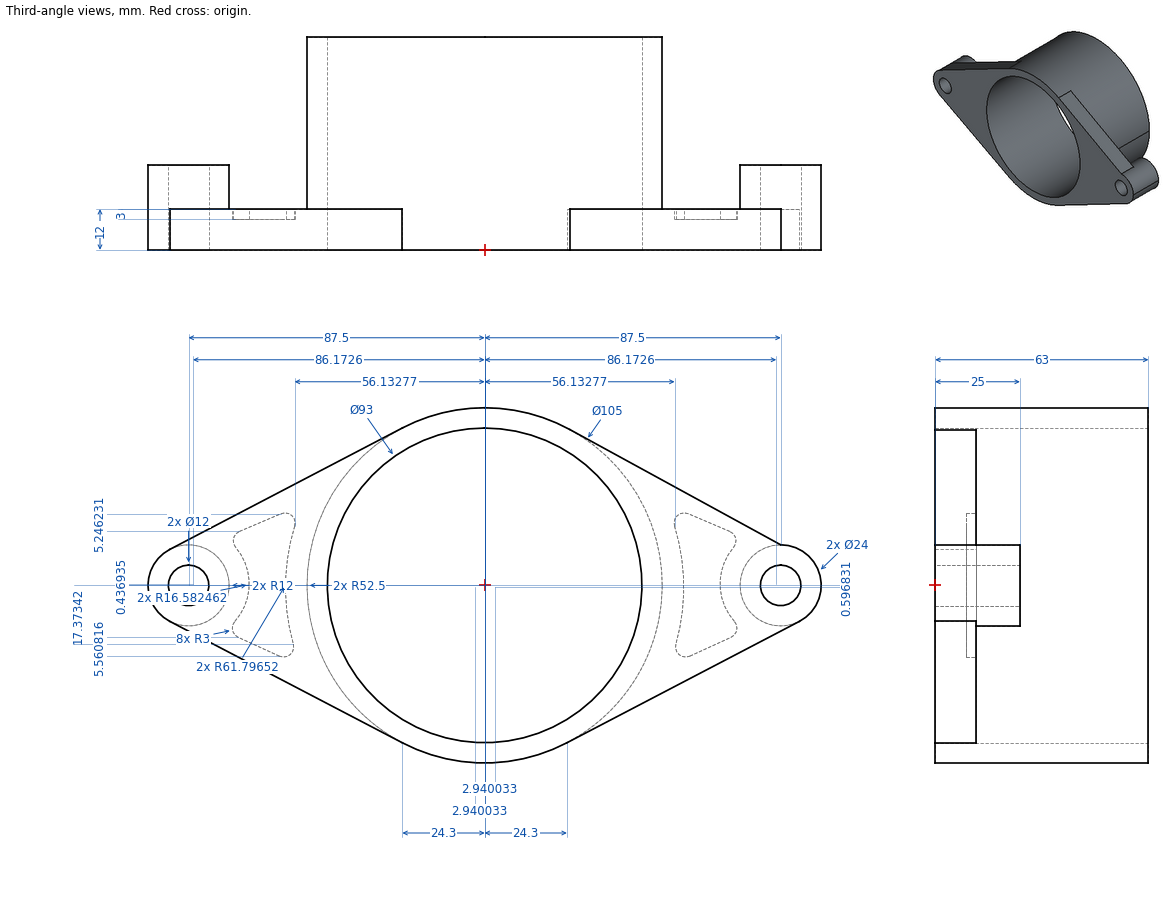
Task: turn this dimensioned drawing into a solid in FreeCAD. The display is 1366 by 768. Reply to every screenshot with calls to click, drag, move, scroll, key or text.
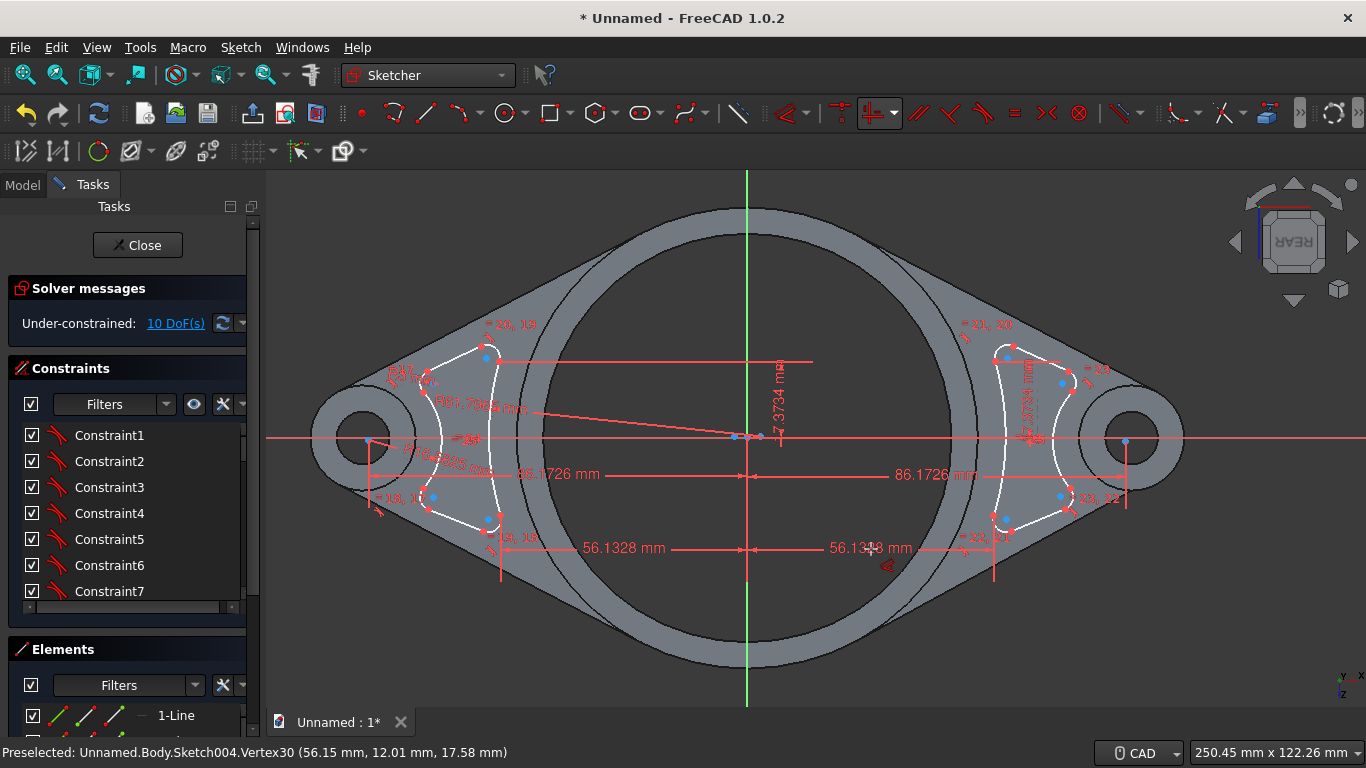
scroll(465, 354, up, 3)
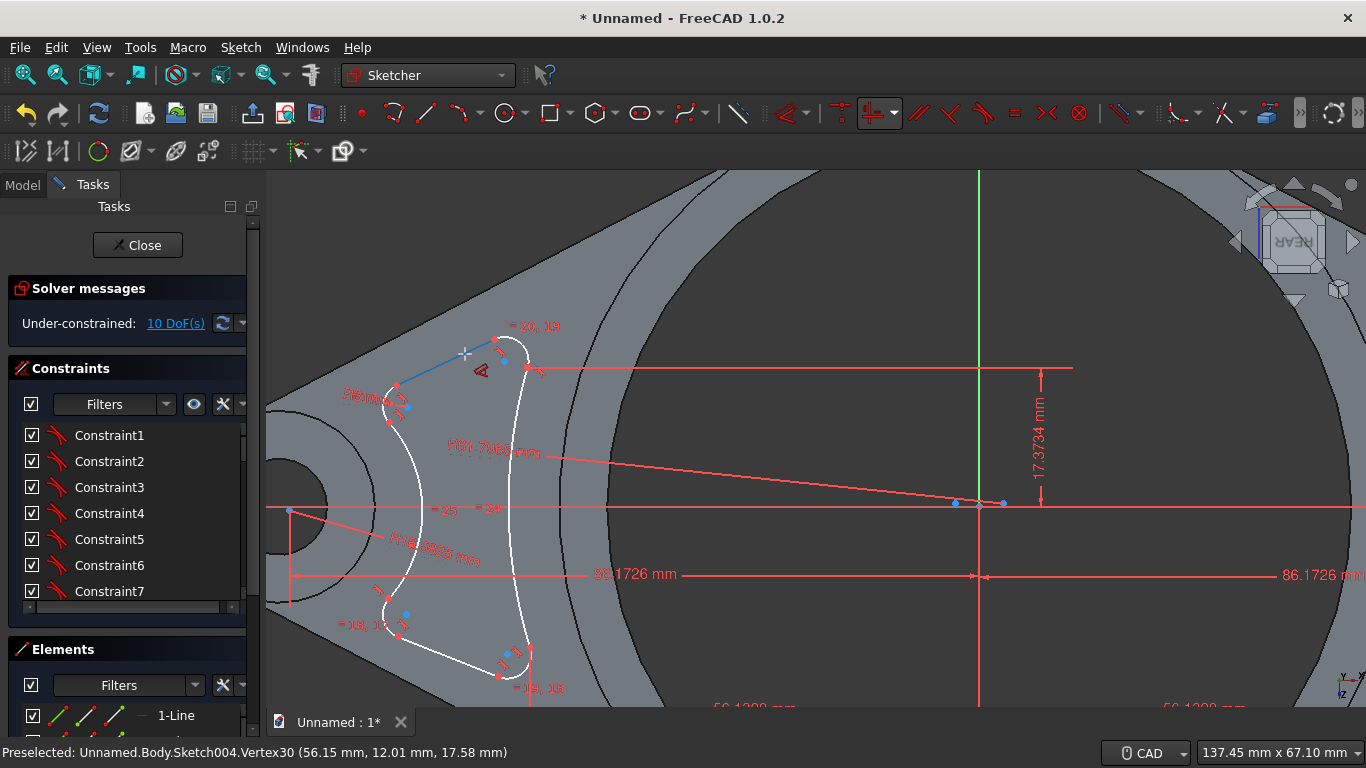
click(465, 353)
click(363, 362)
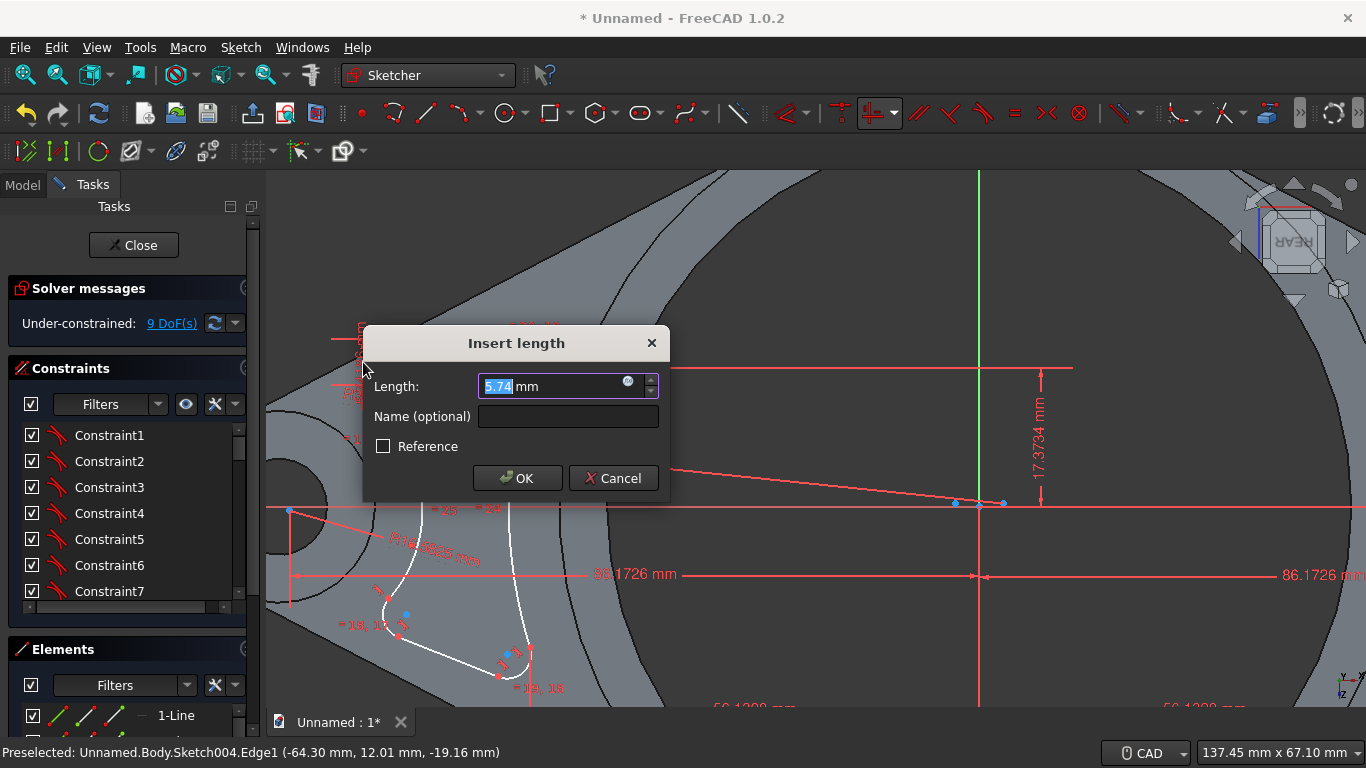
text(5.560816)
key(Return)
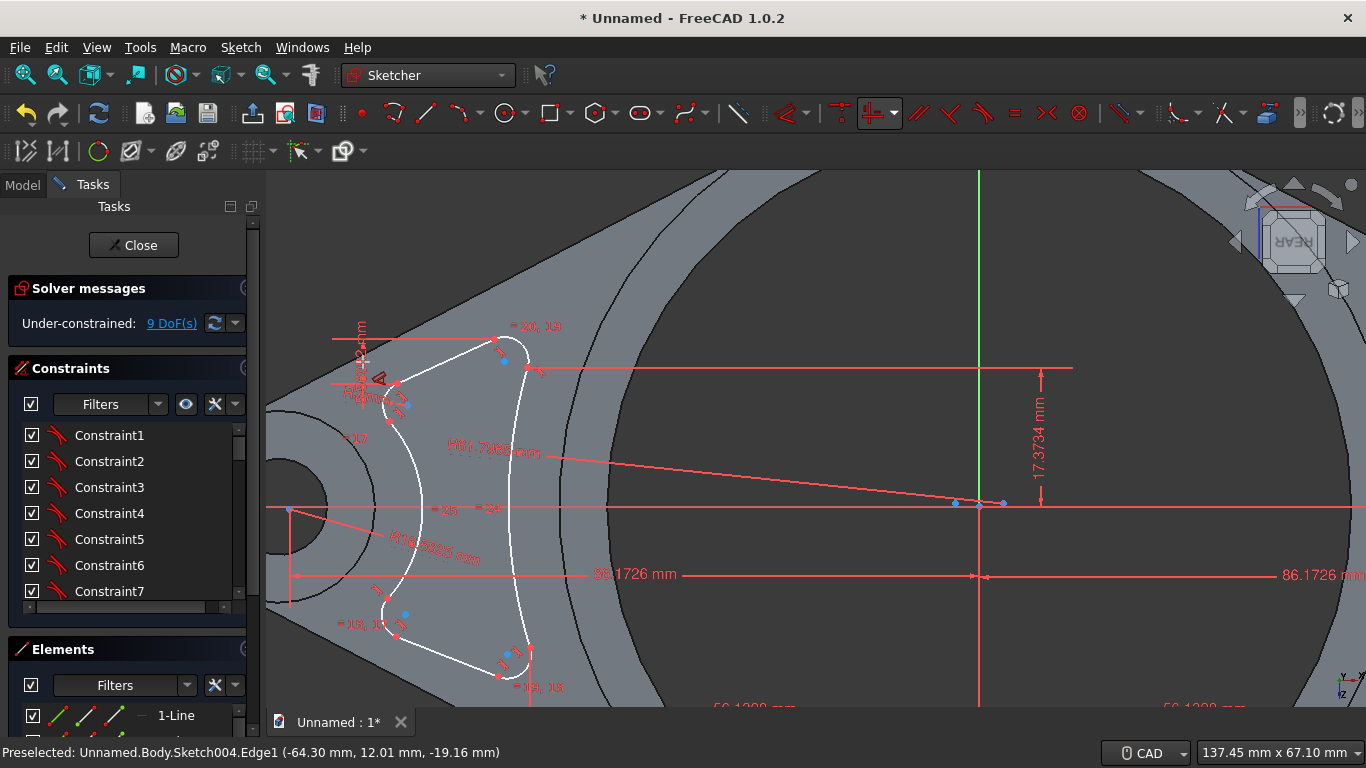
click(427, 649)
click(363, 657)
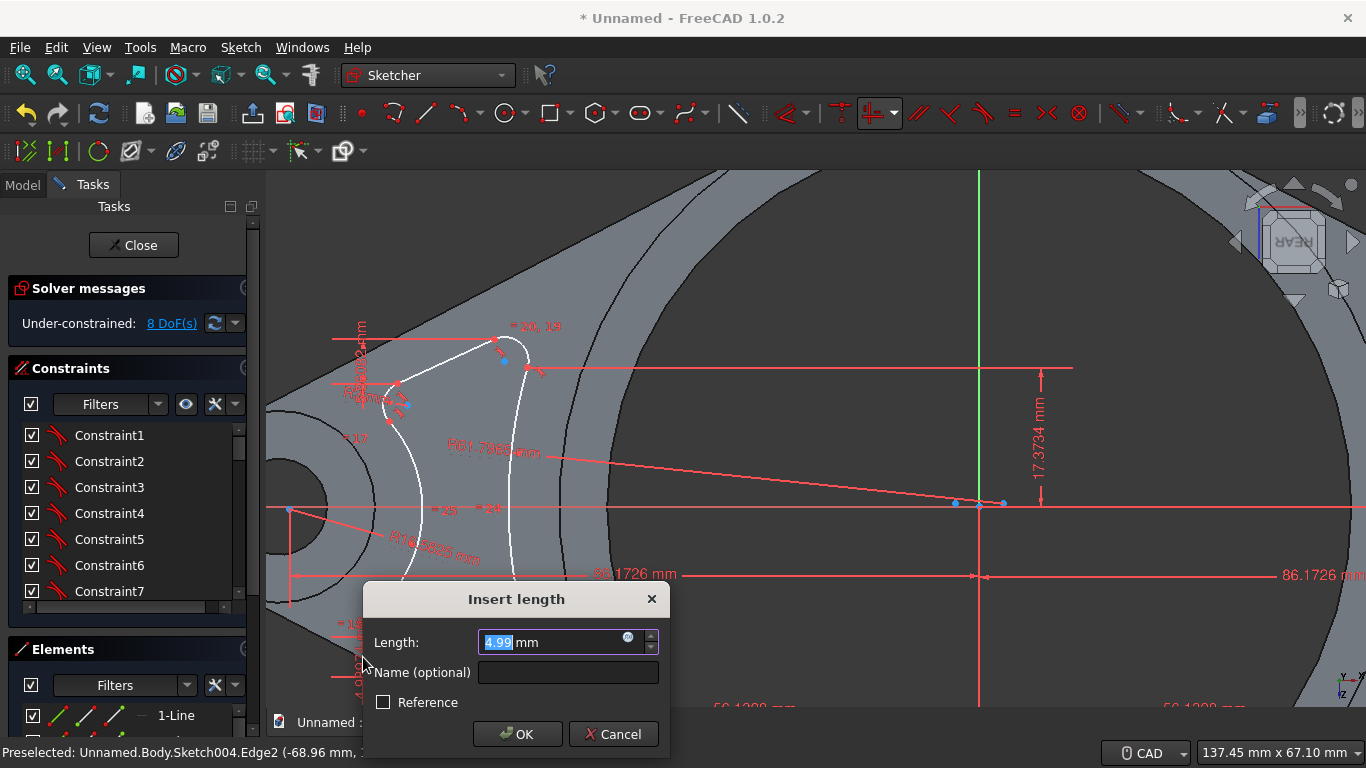
text(5.246231)
key(Return)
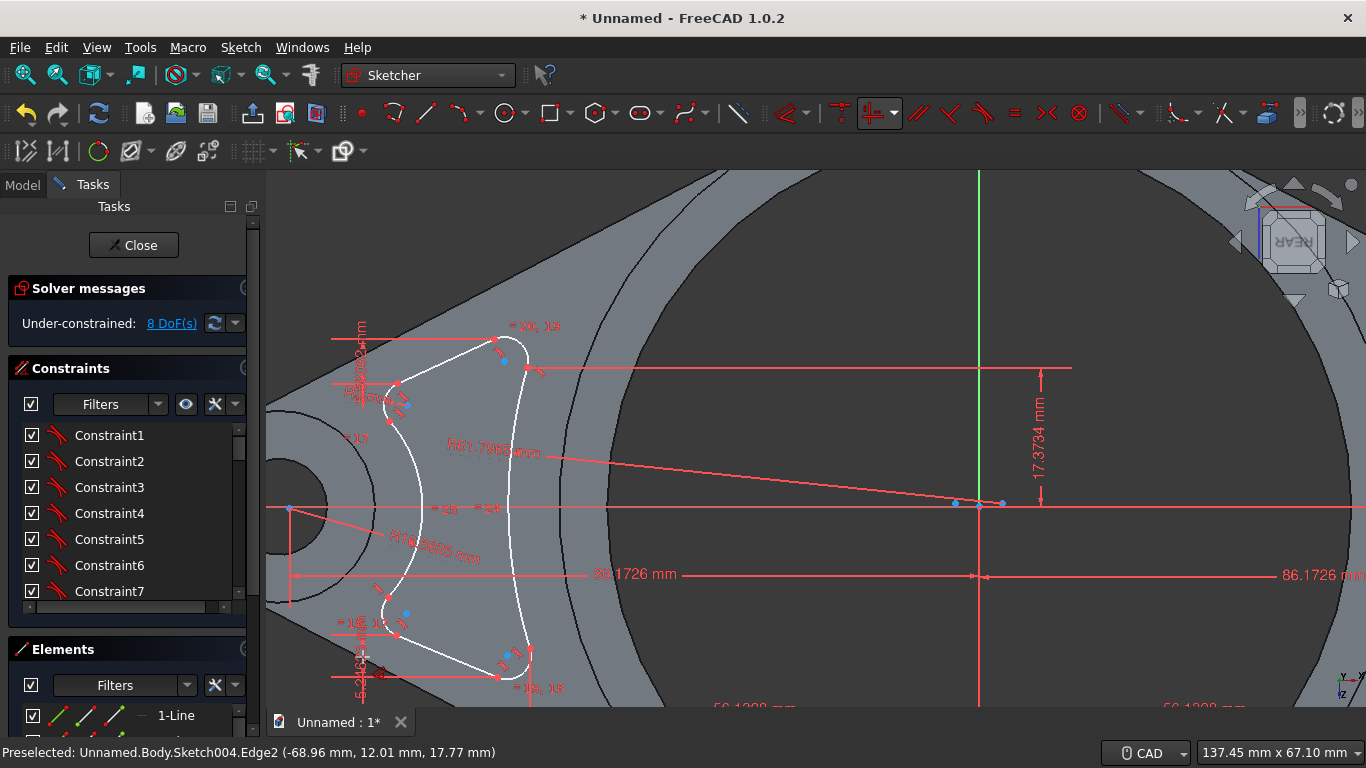
scroll(466, 354, down, 3)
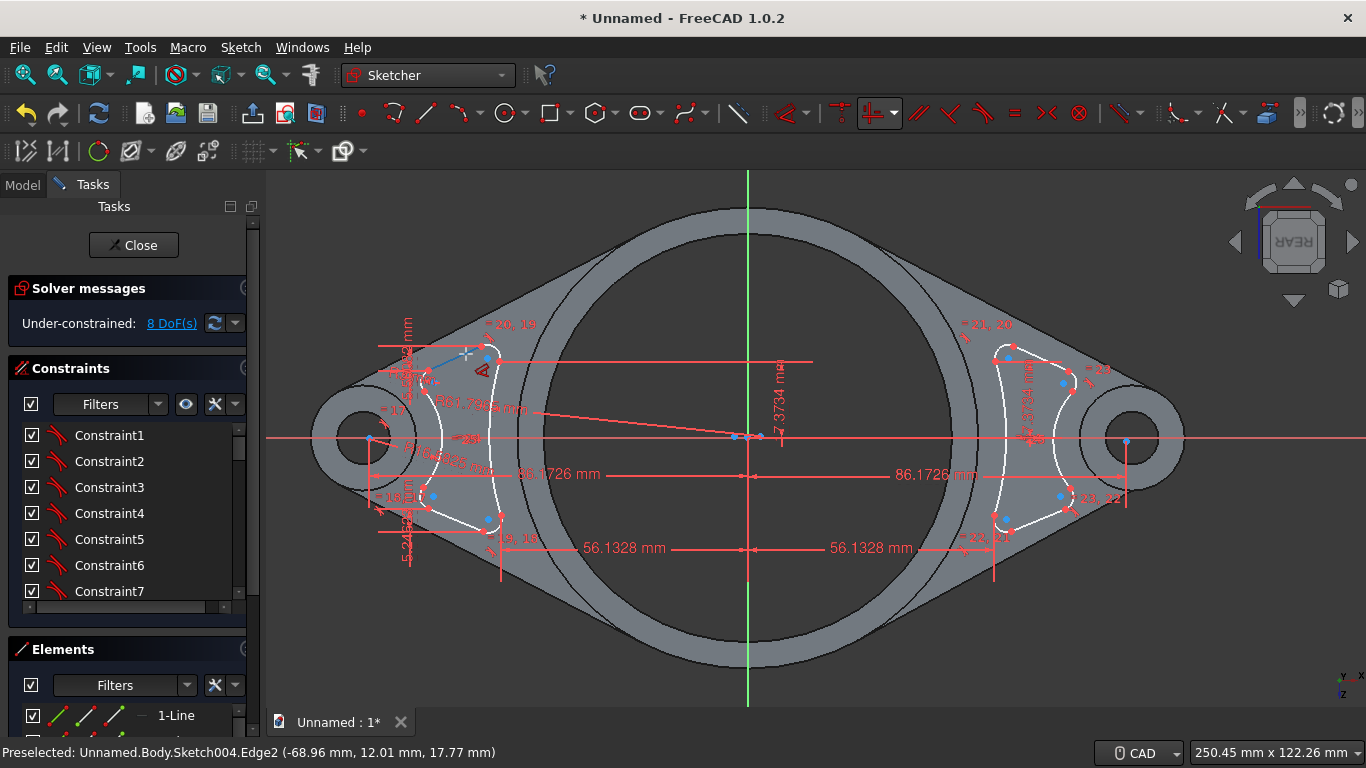
scroll(1052, 364, up, 3)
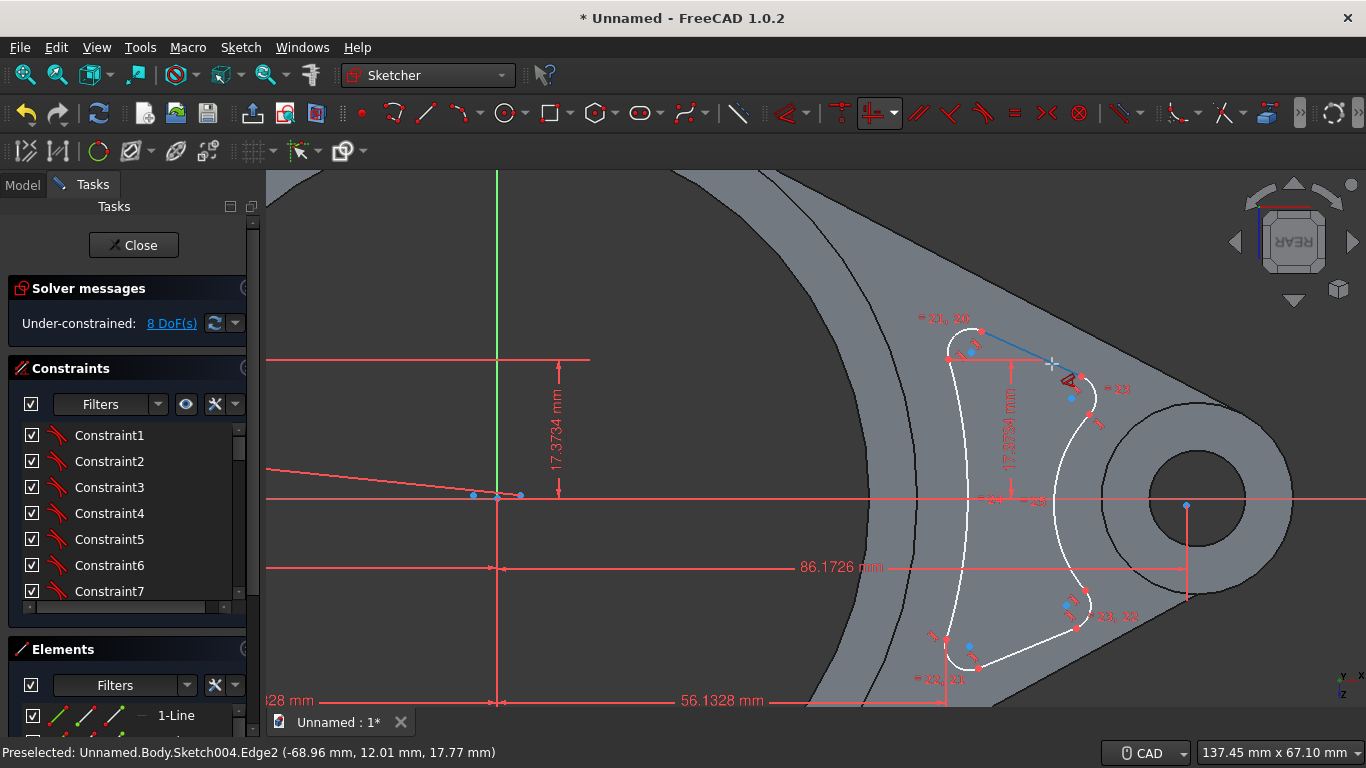
click(1052, 363)
click(1116, 354)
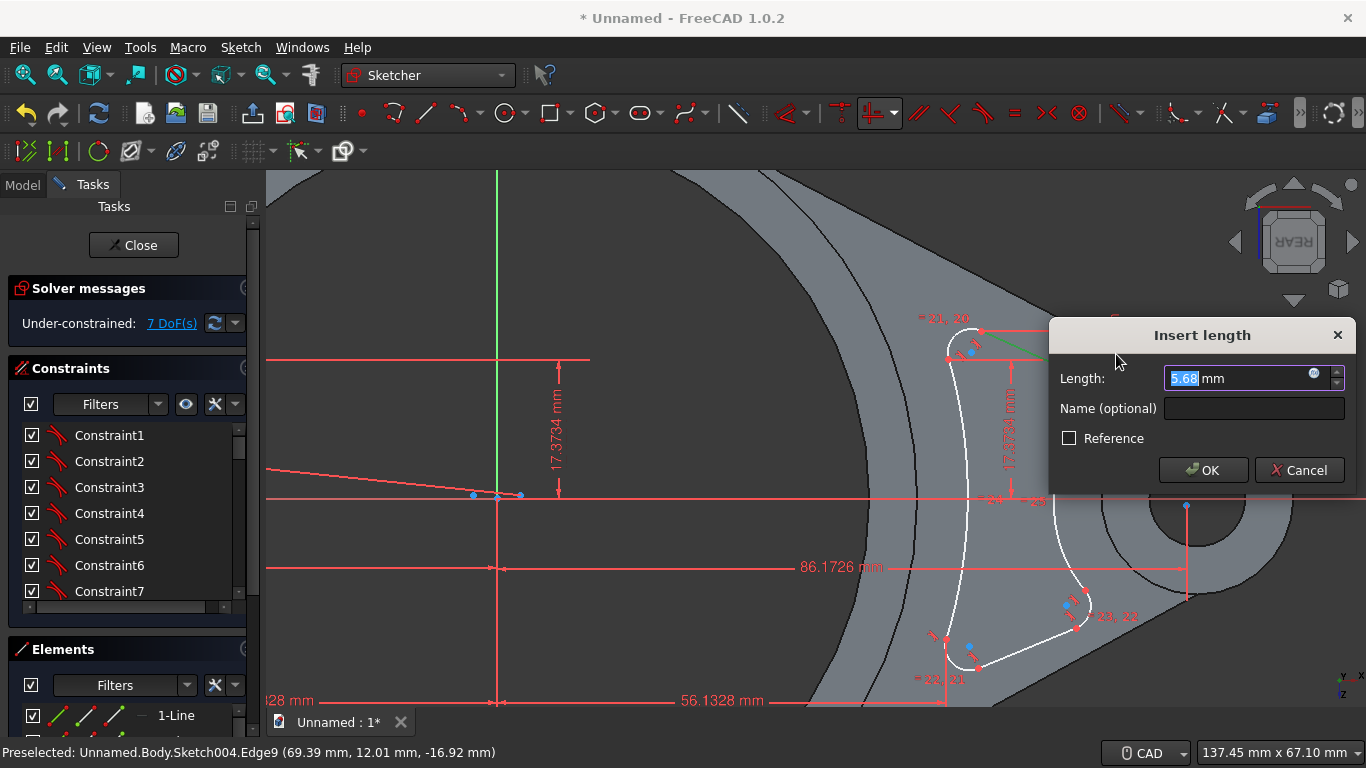
text(5.560816)
key(Return)